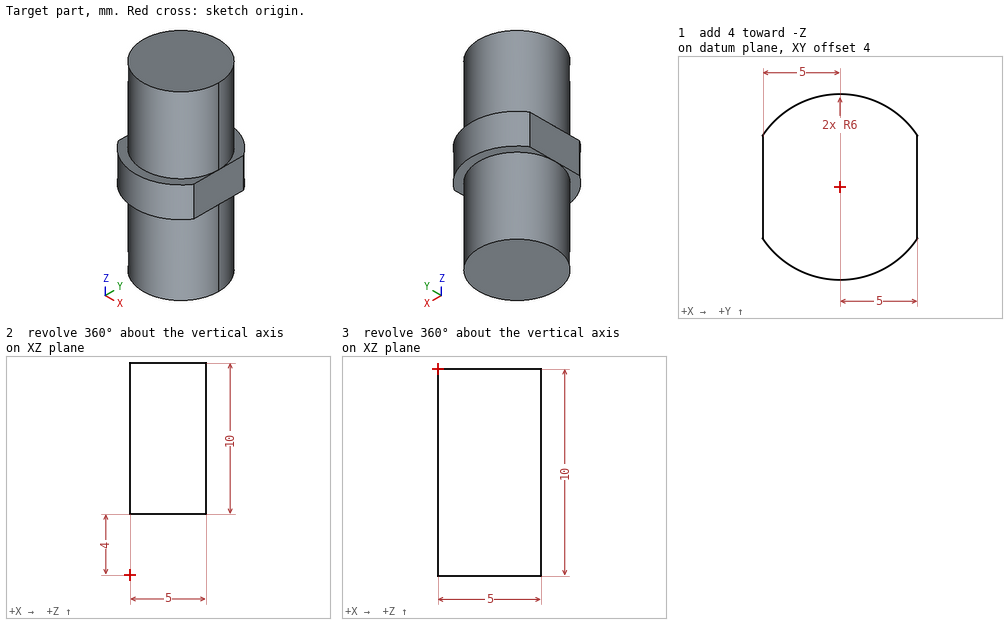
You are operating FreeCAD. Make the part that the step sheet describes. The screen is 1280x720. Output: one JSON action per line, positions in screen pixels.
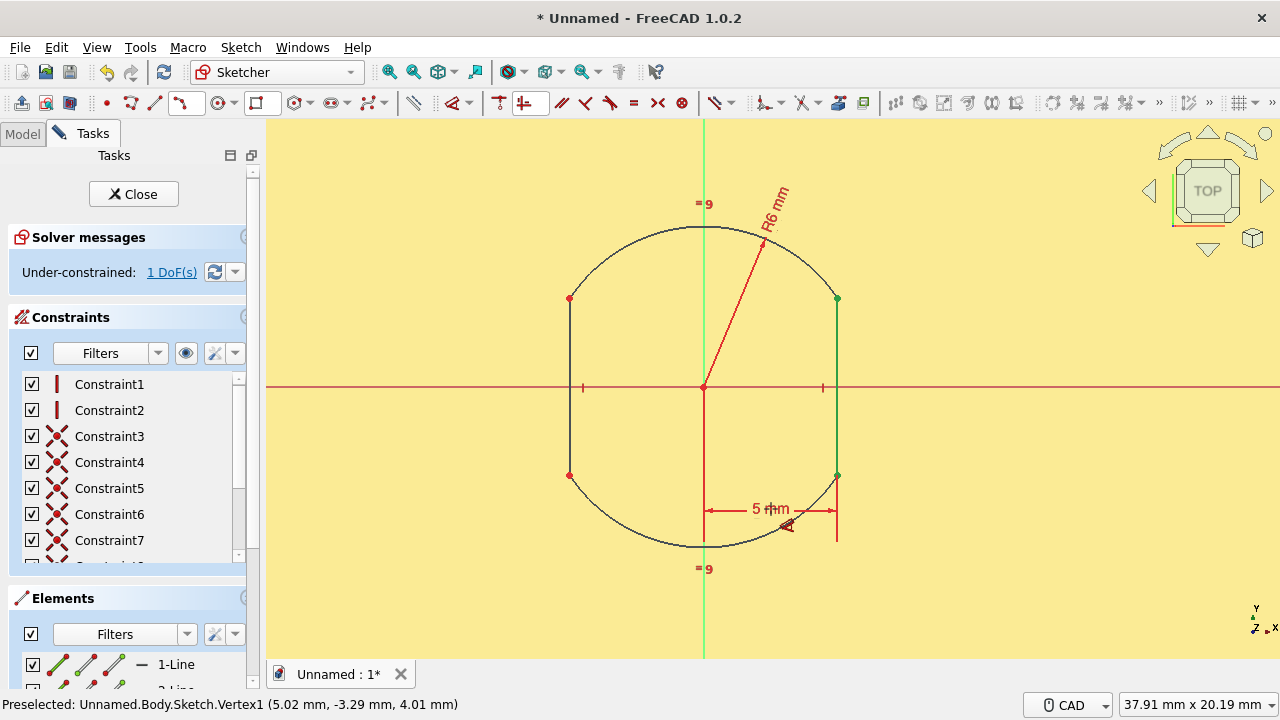
{"action": "left_click", "coordinate": [570, 299]}
{"action": "left_click", "coordinate": [637, 265]}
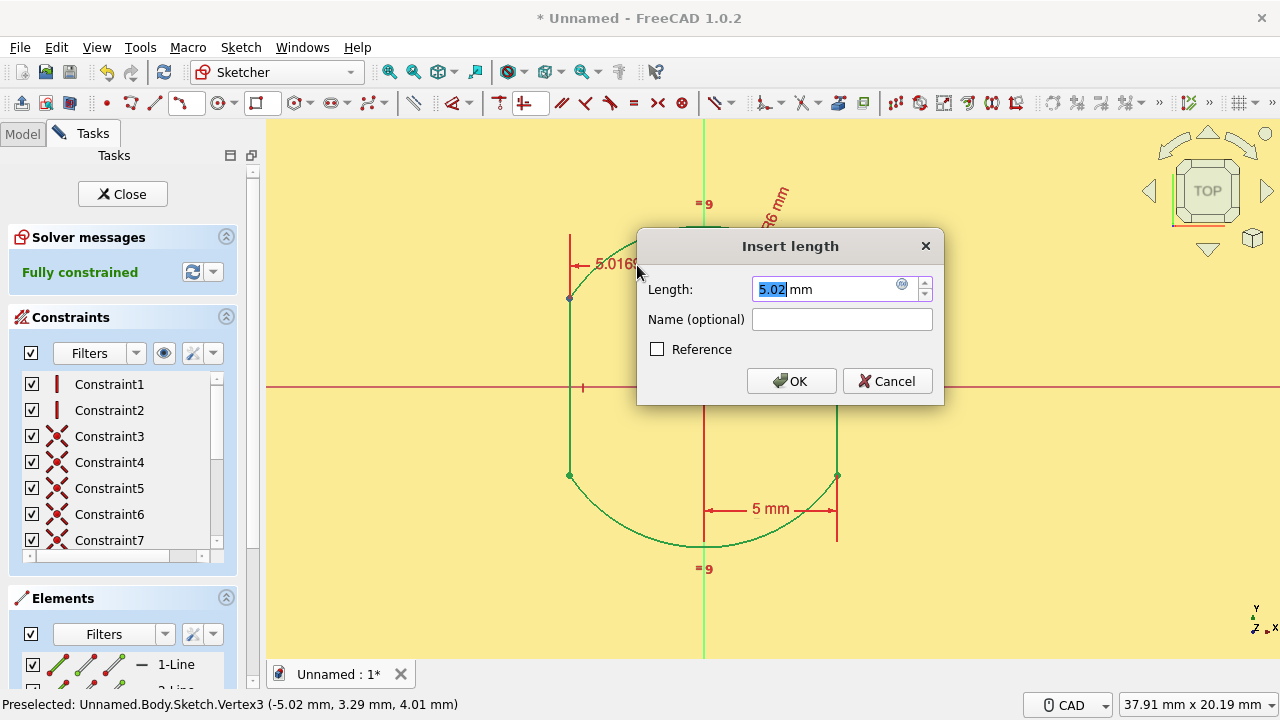
{"action": "type", "text": "5"}
{"action": "key", "text": "Return"}
{"action": "key", "text": "Escape"}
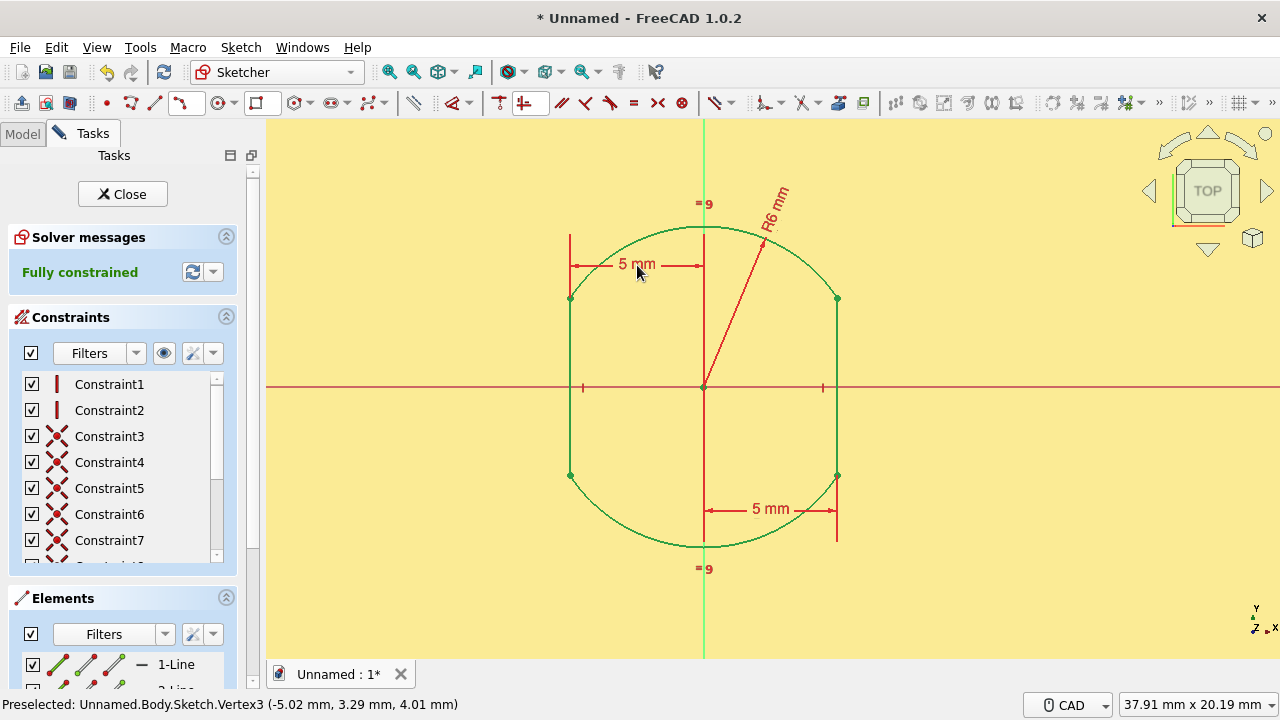
{"action": "left_click", "coordinate": [123, 194]}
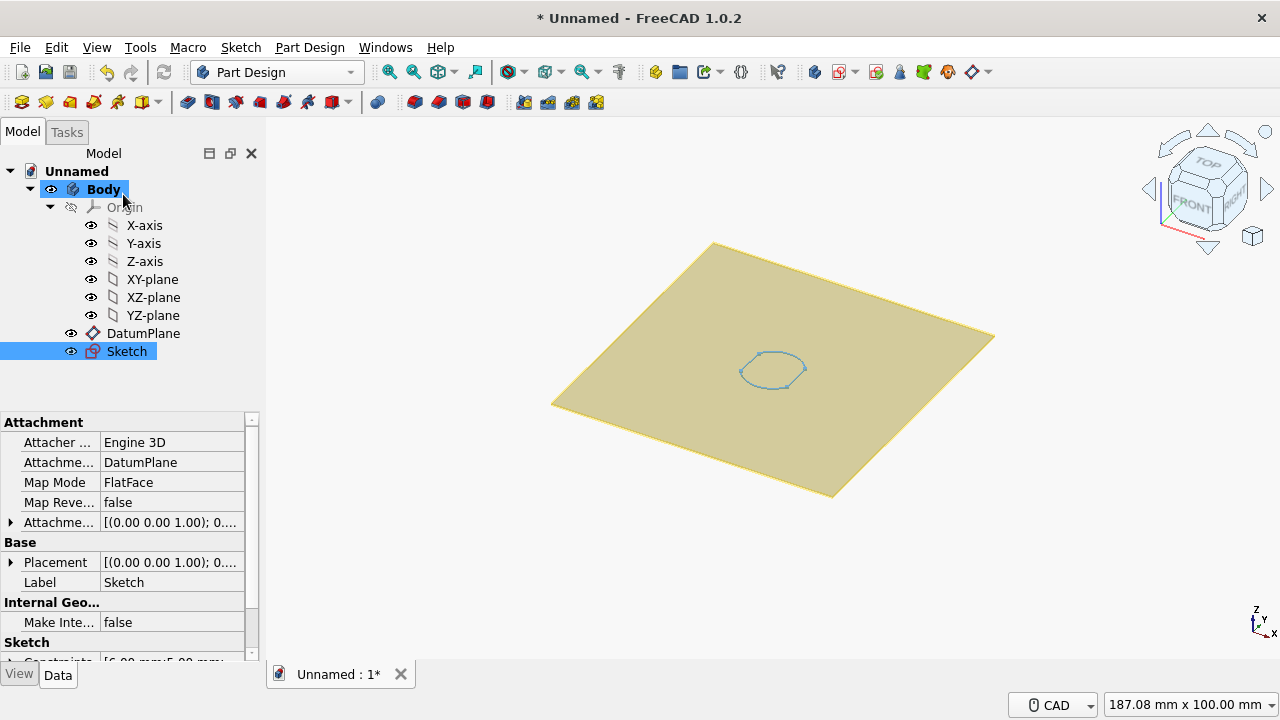
{"action": "left_click", "coordinate": [22, 102]}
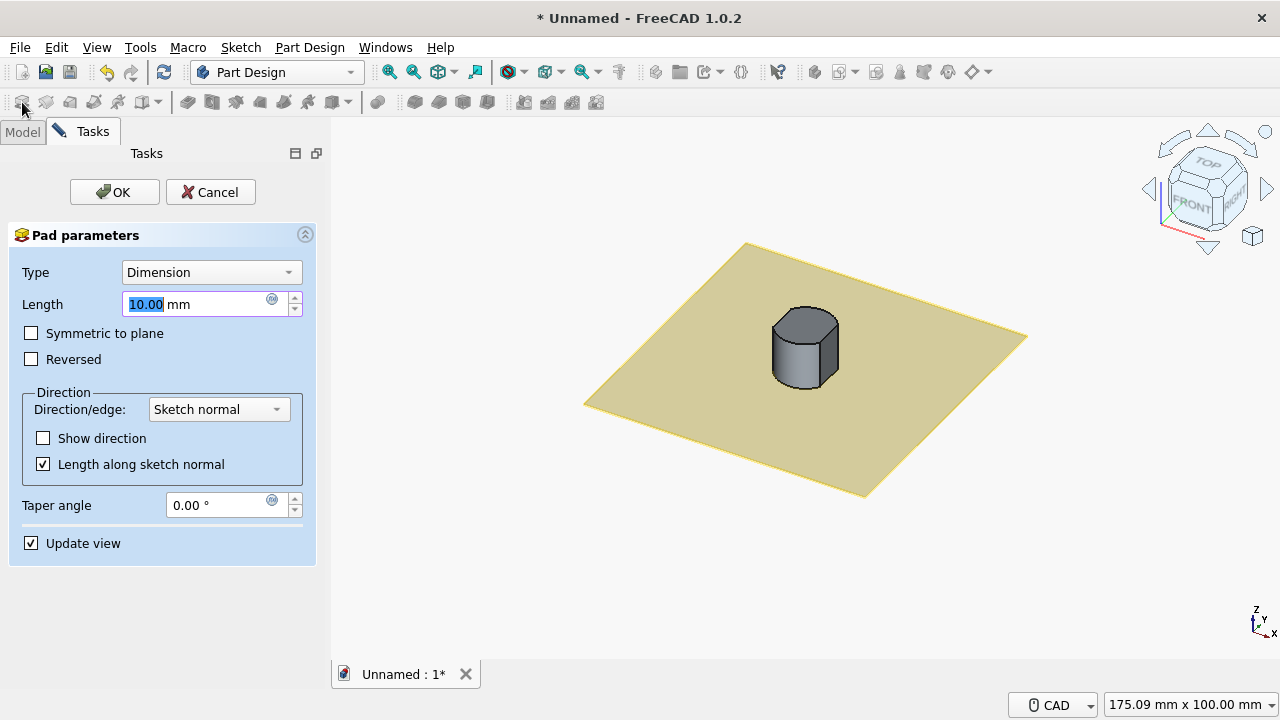
{"action": "type", "text": "4"}
{"action": "key", "text": "Tab"}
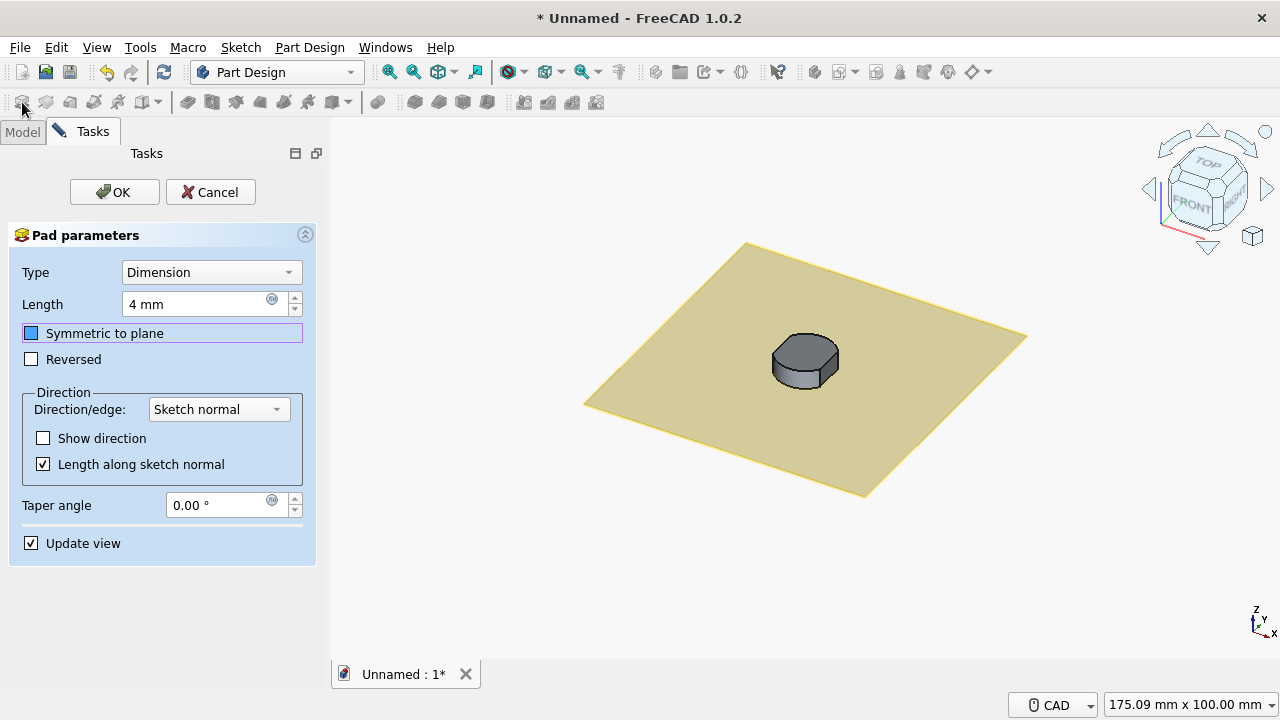
{"action": "left_click", "coordinate": [30, 359]}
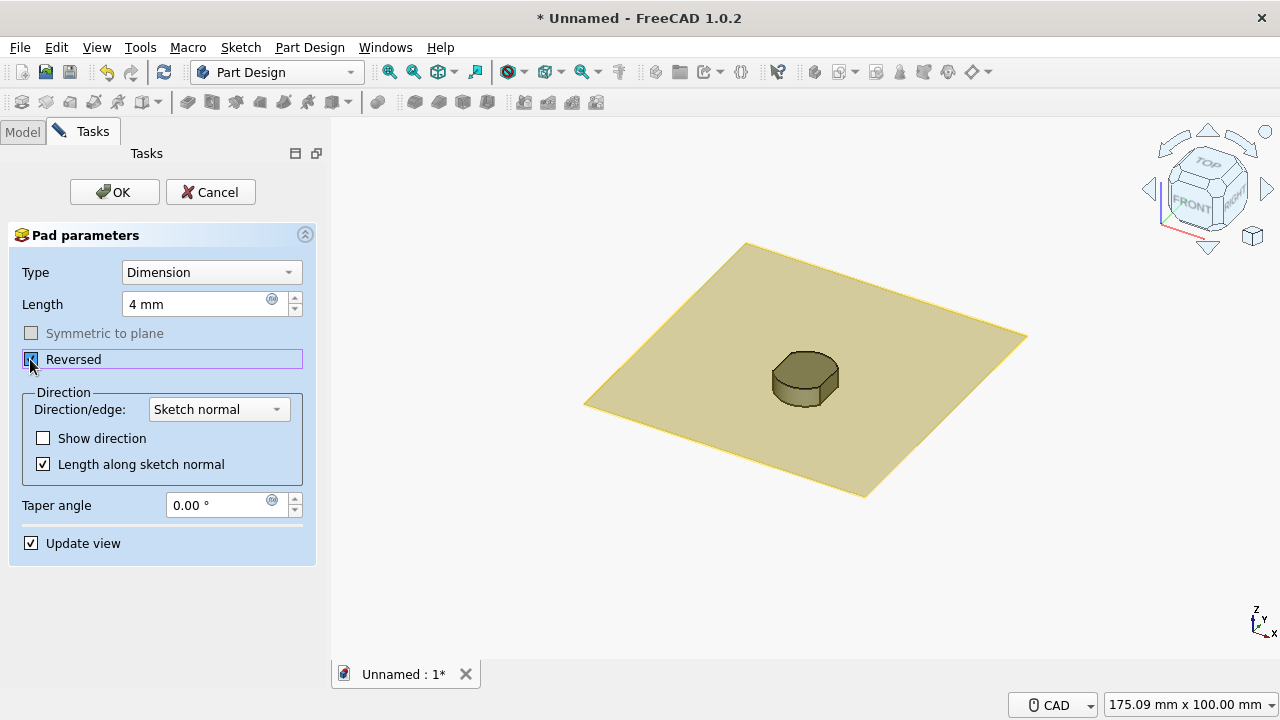
{"action": "left_click", "coordinate": [115, 192]}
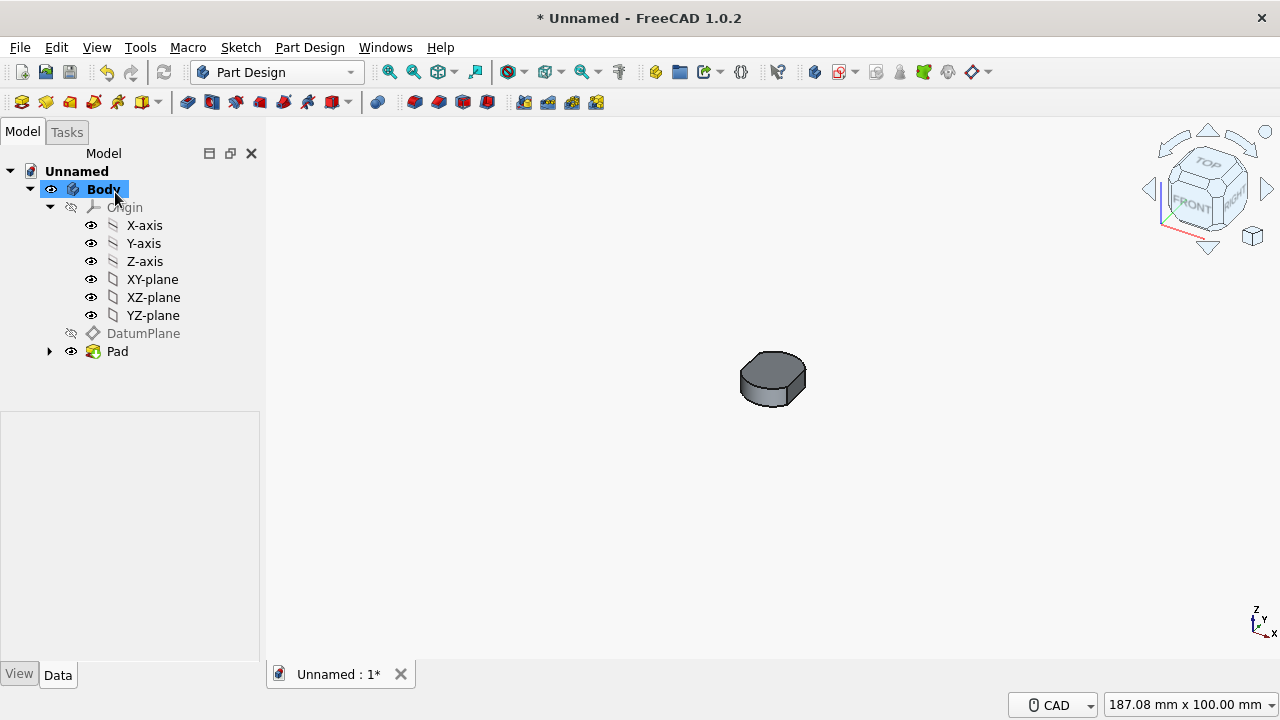
{"action": "key", "text": "v f"}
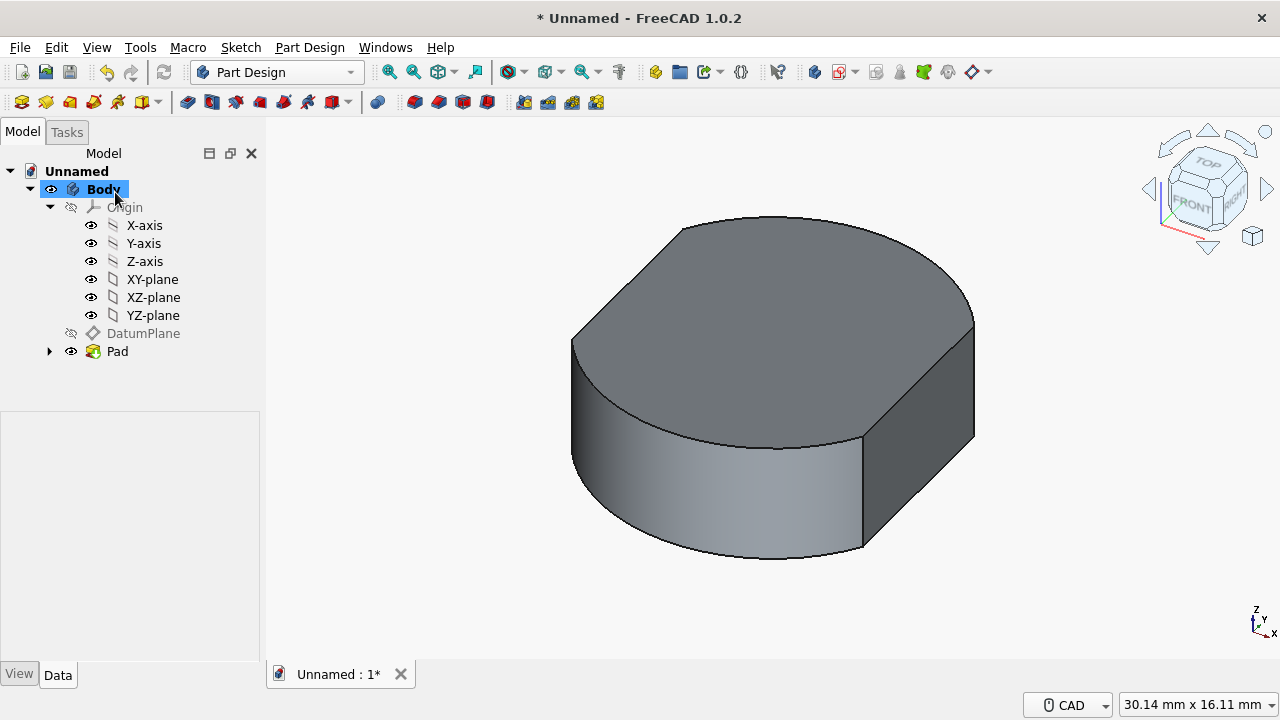
{"action": "left_click", "coordinate": [840, 72]}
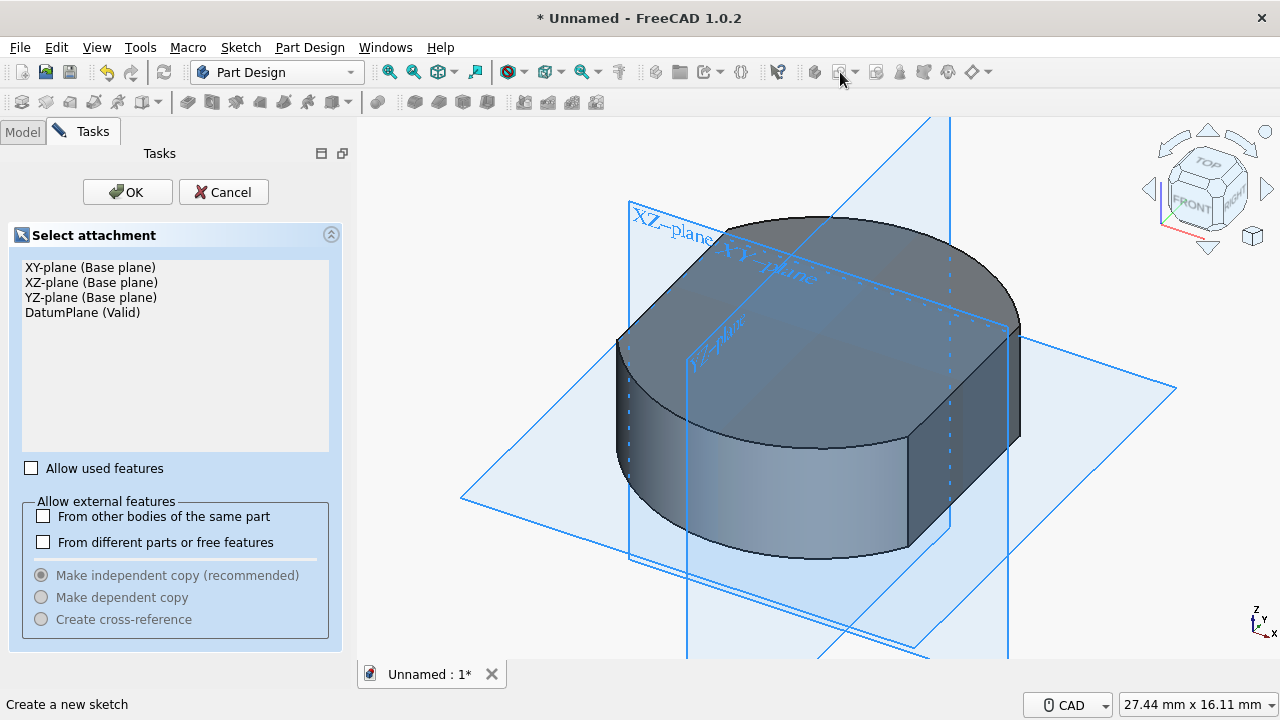
{"action": "left_click", "coordinate": [82, 282]}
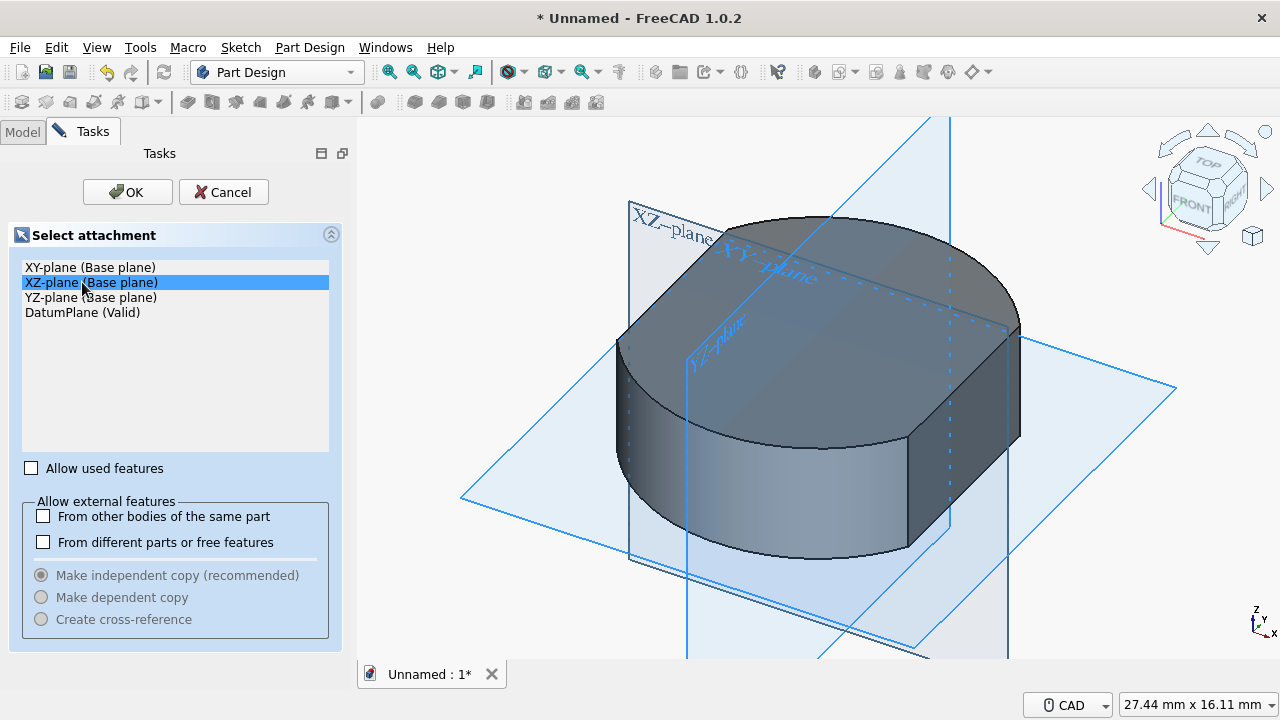
{"action": "left_click", "coordinate": [128, 192]}